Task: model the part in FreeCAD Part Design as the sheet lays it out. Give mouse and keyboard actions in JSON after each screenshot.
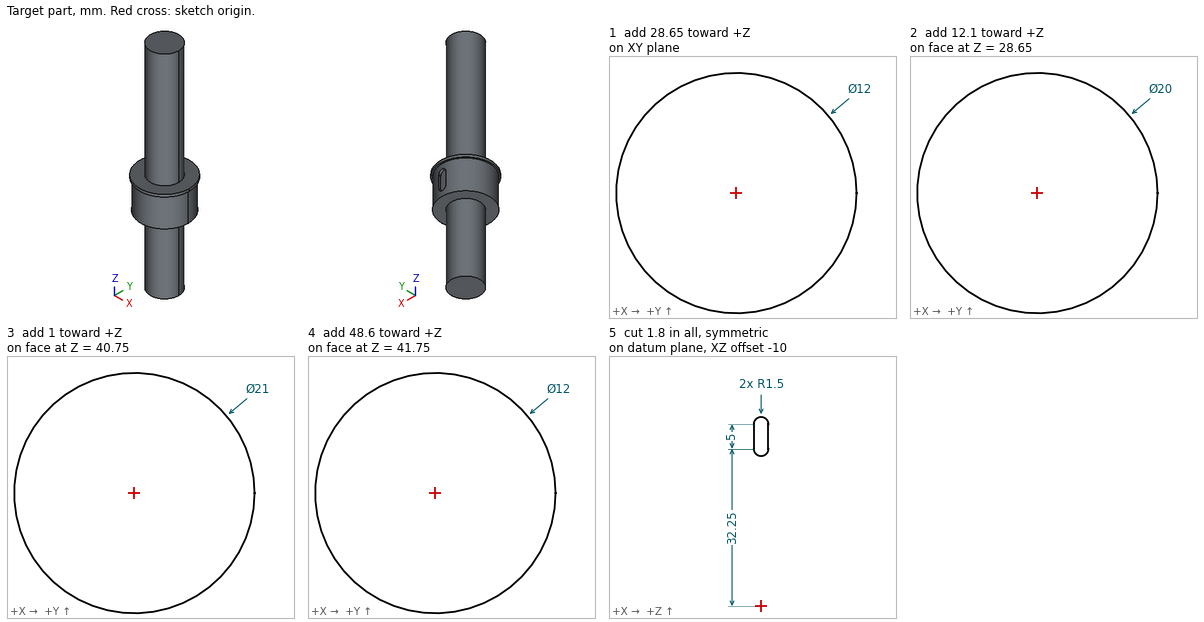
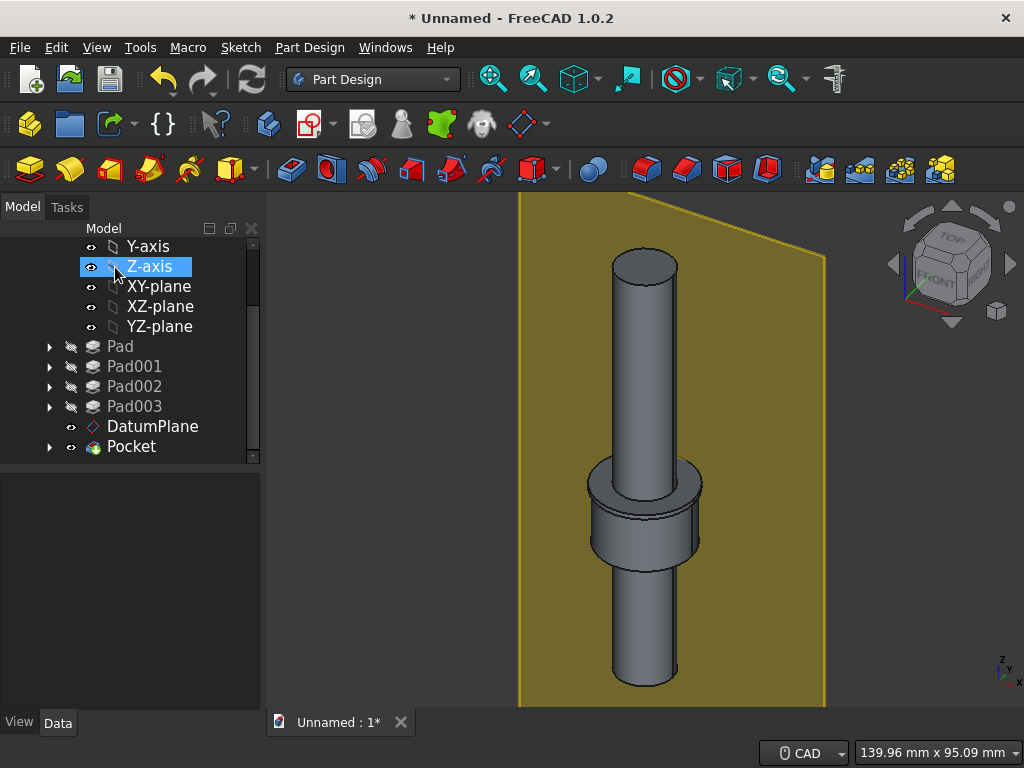
{"action": "left_click", "coordinate": [116, 427]}
{"action": "key", "text": "space"}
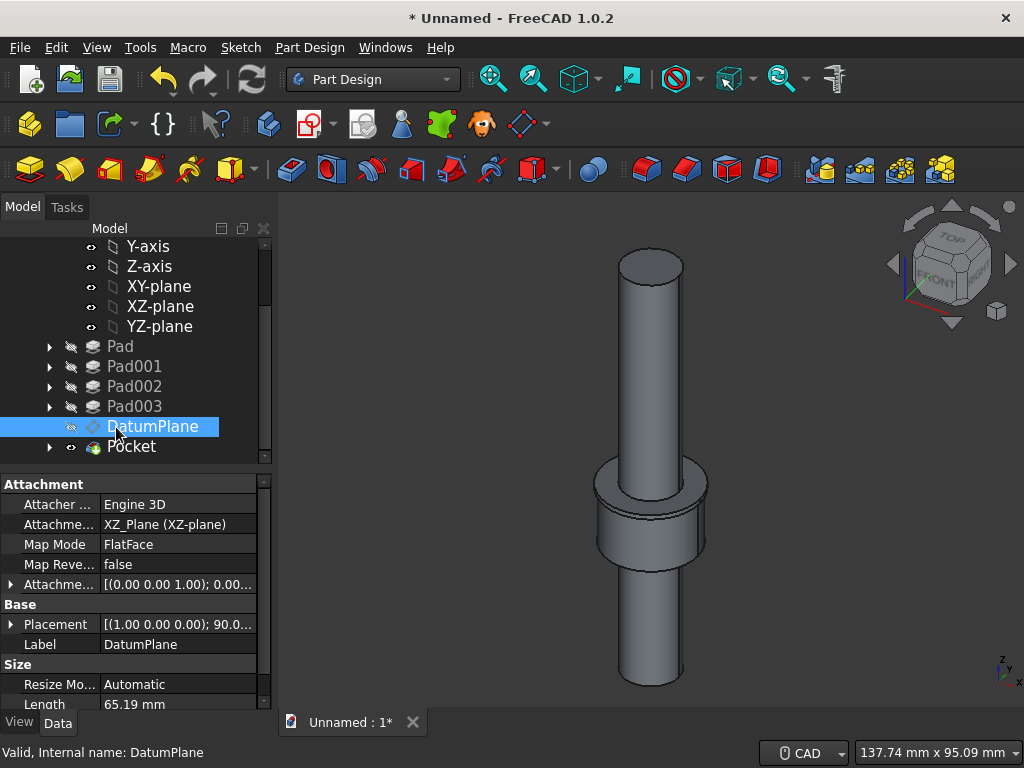
{"action": "key", "text": "0"}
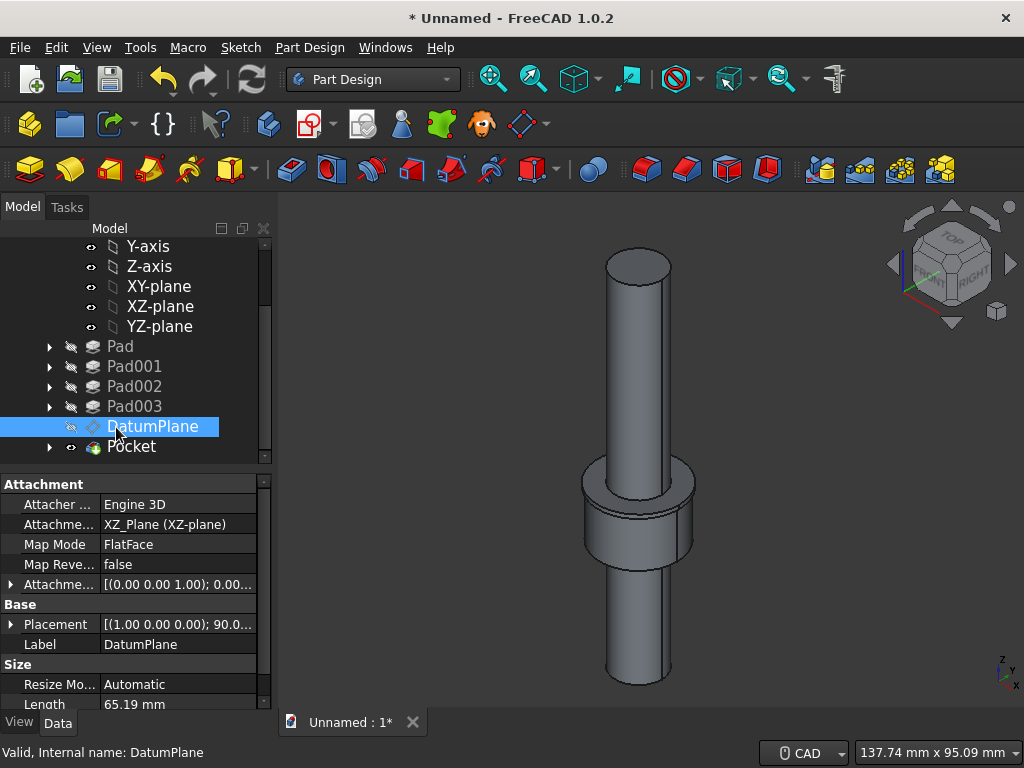
{"action": "left_click", "coordinate": [494, 80]}